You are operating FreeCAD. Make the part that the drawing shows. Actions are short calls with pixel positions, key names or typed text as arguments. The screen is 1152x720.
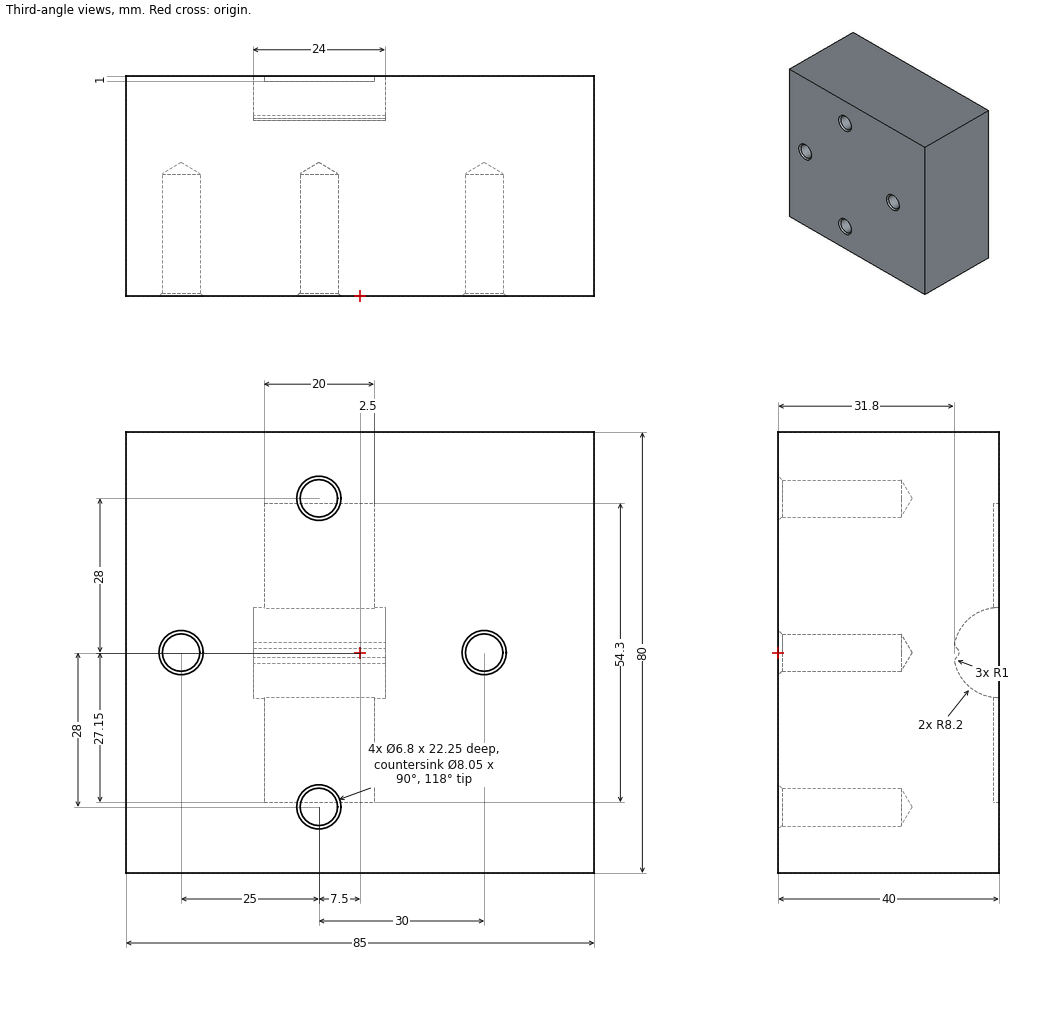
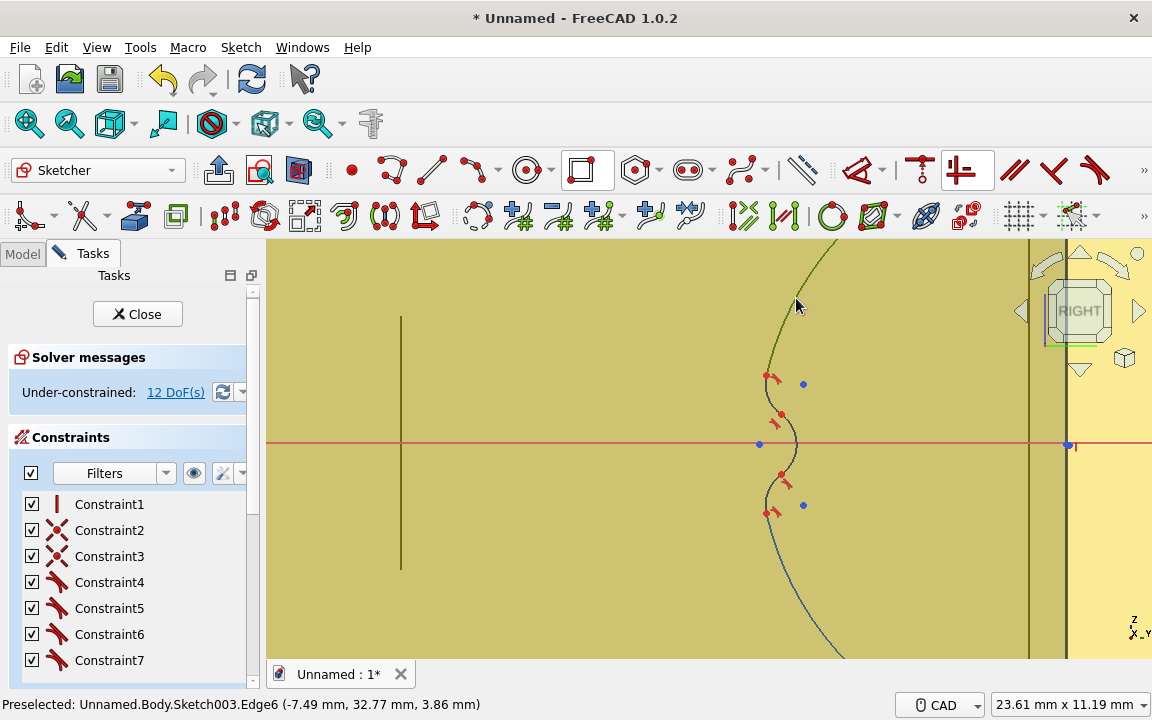
click(920, 170)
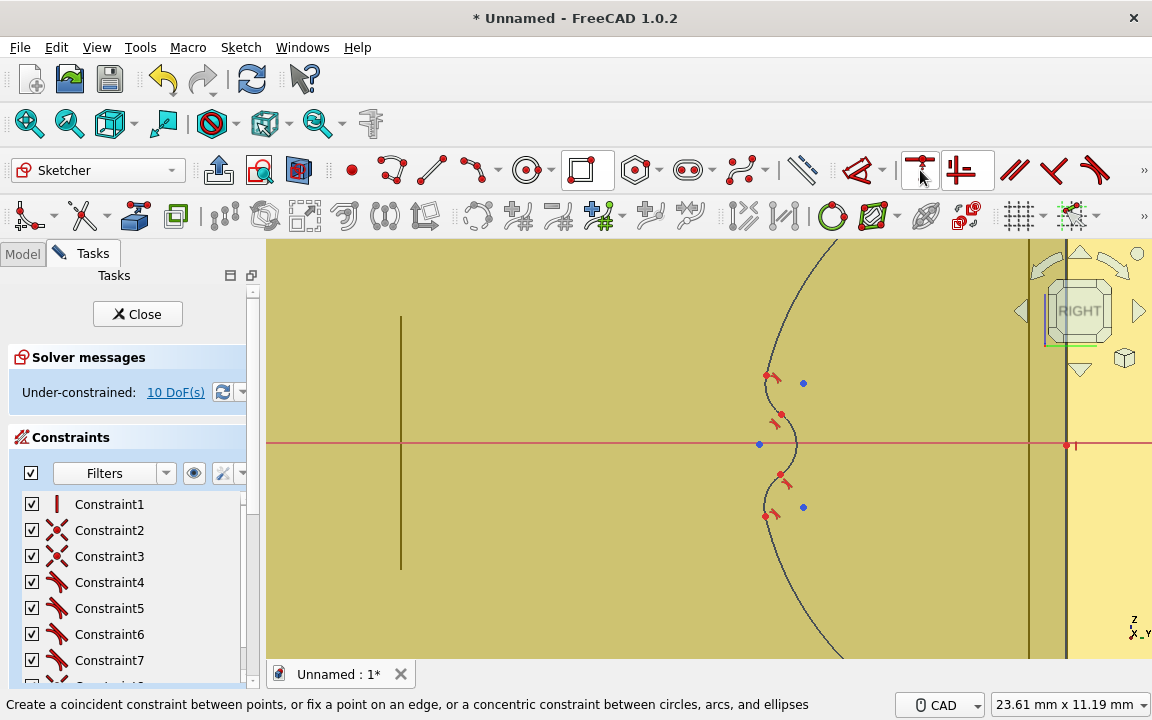
click(771, 485)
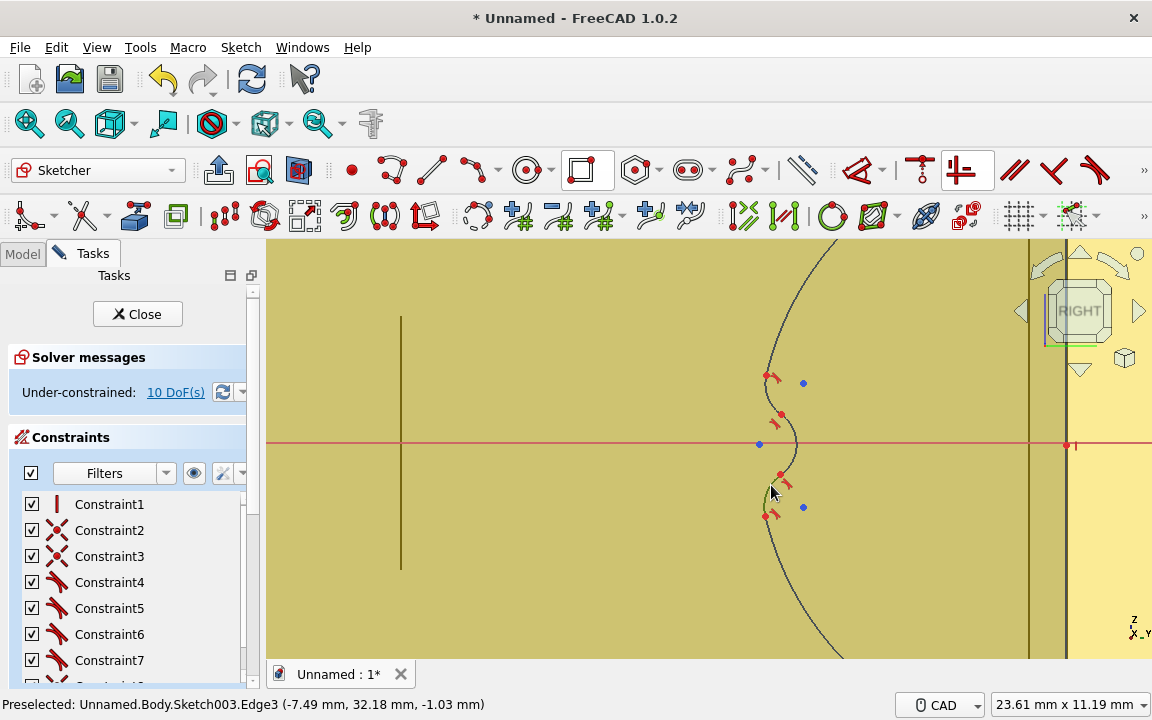
click(794, 458)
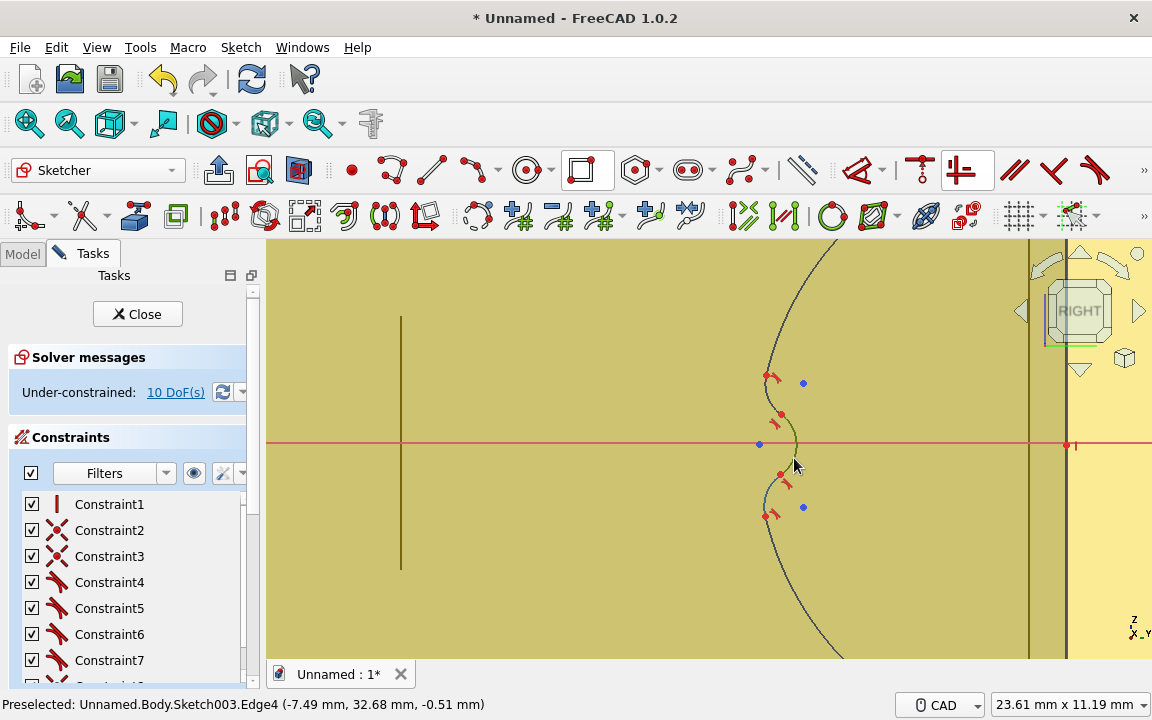
click(766, 389)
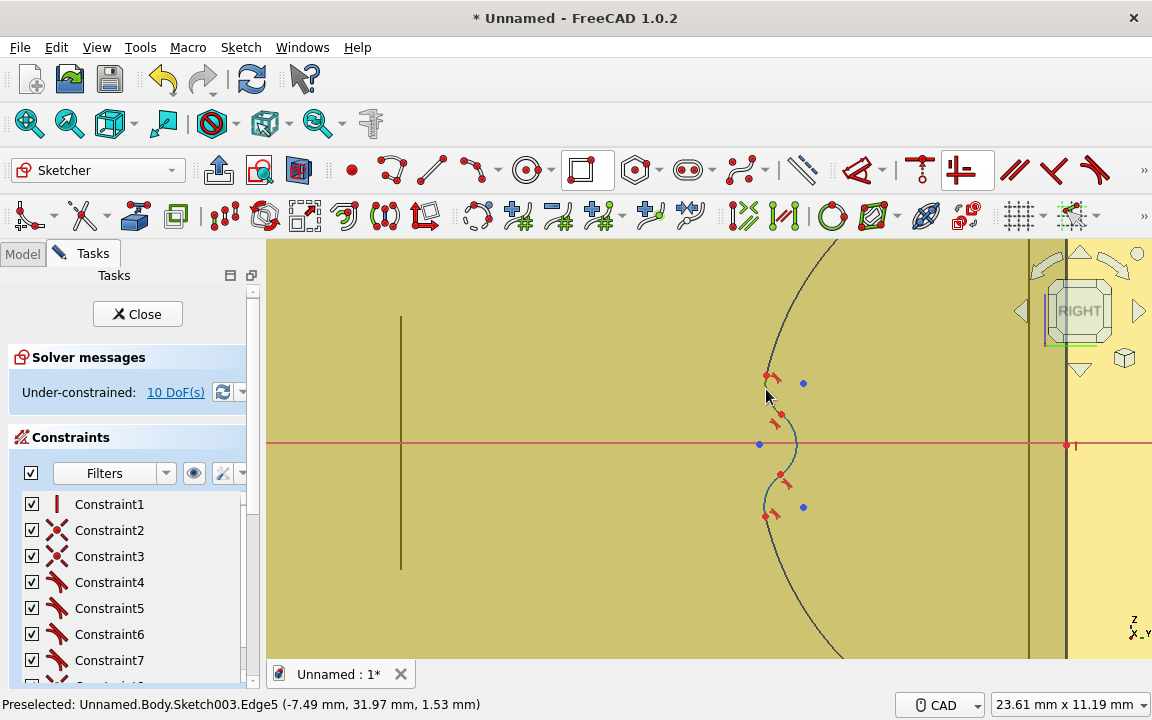
key(e)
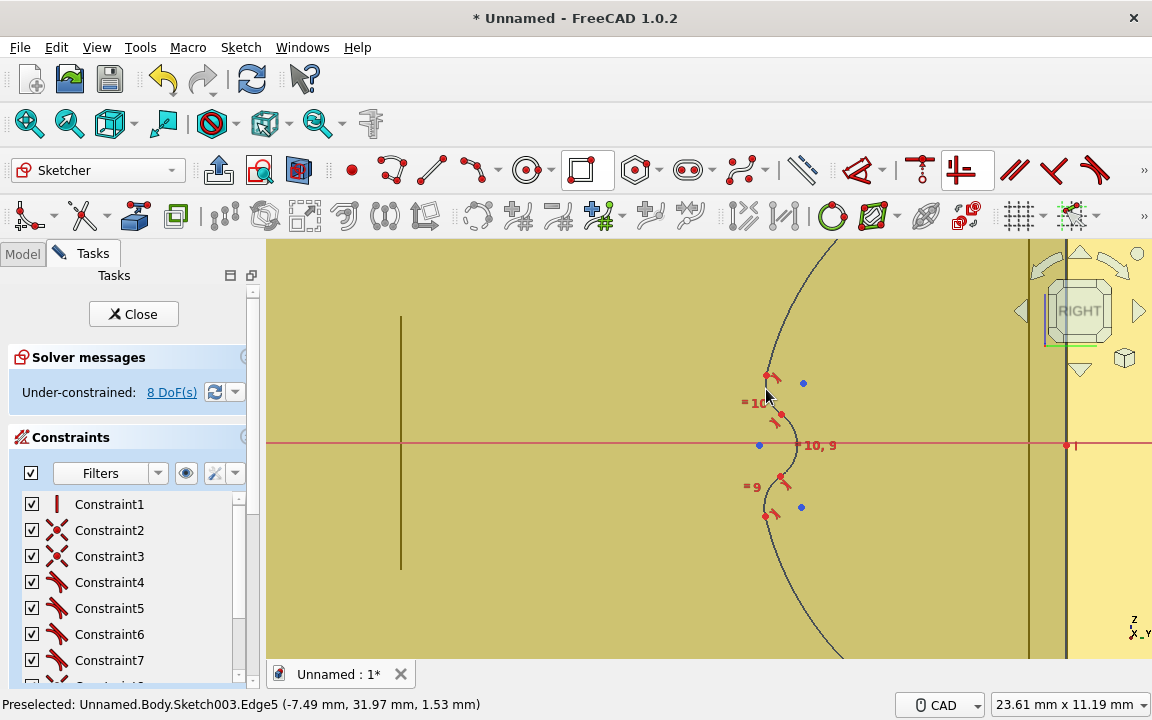
click(817, 628)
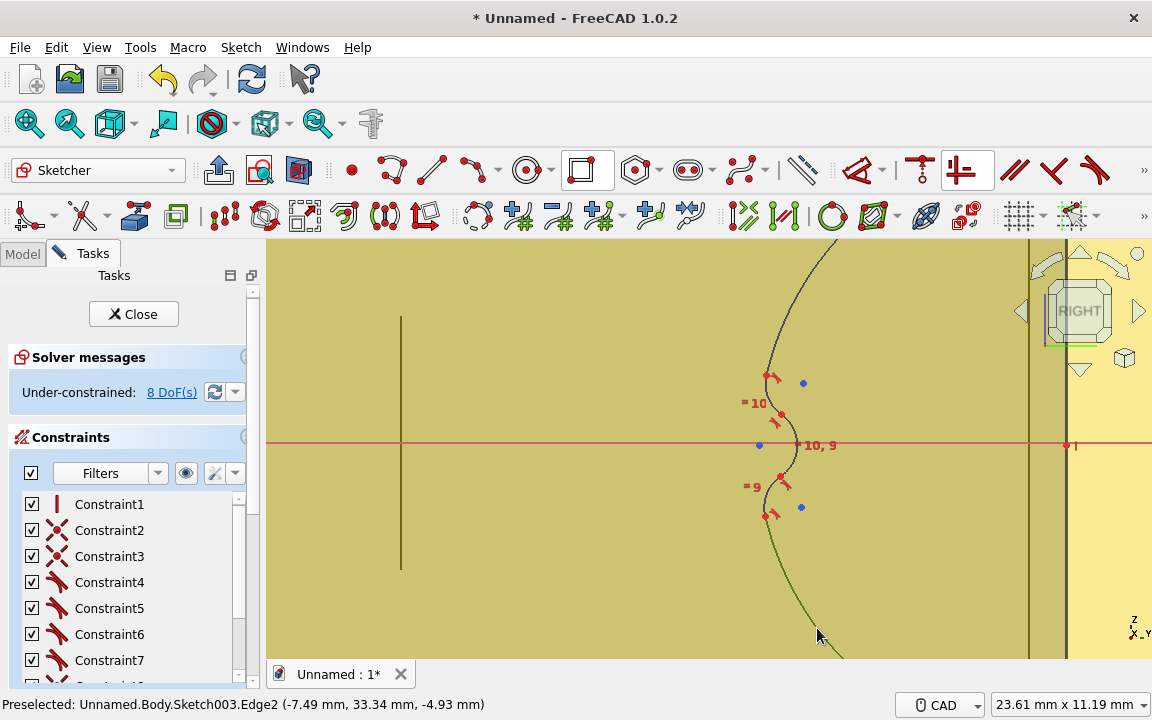
click(796, 298)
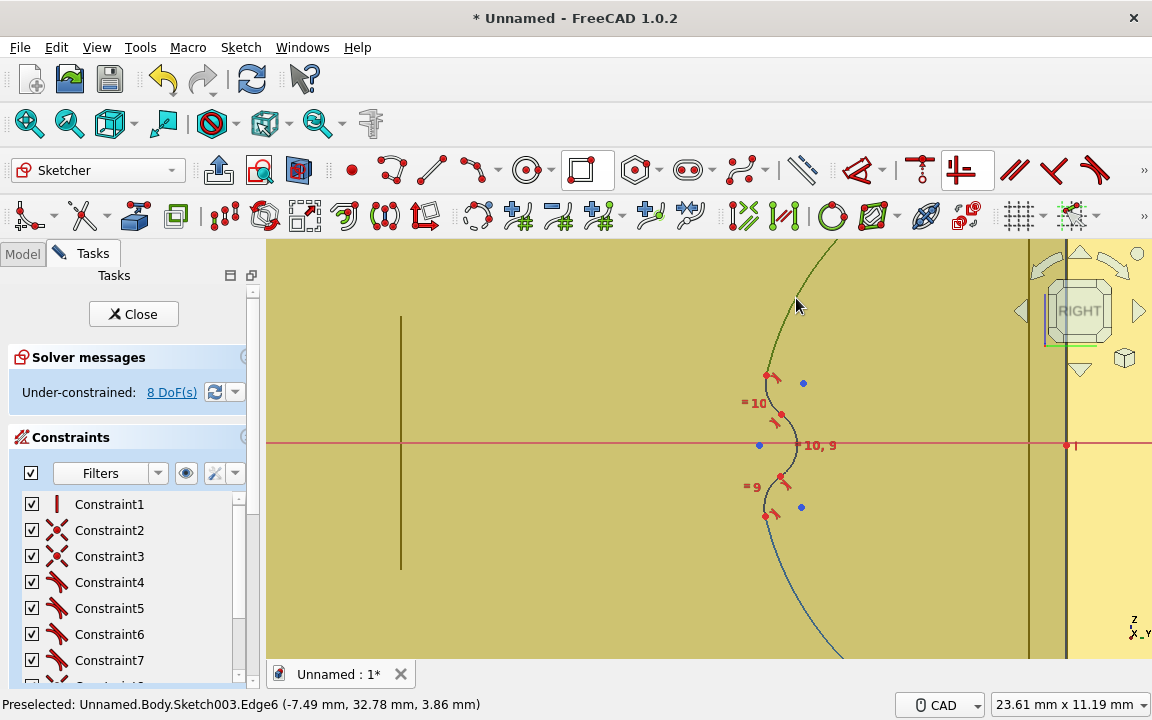
key(e)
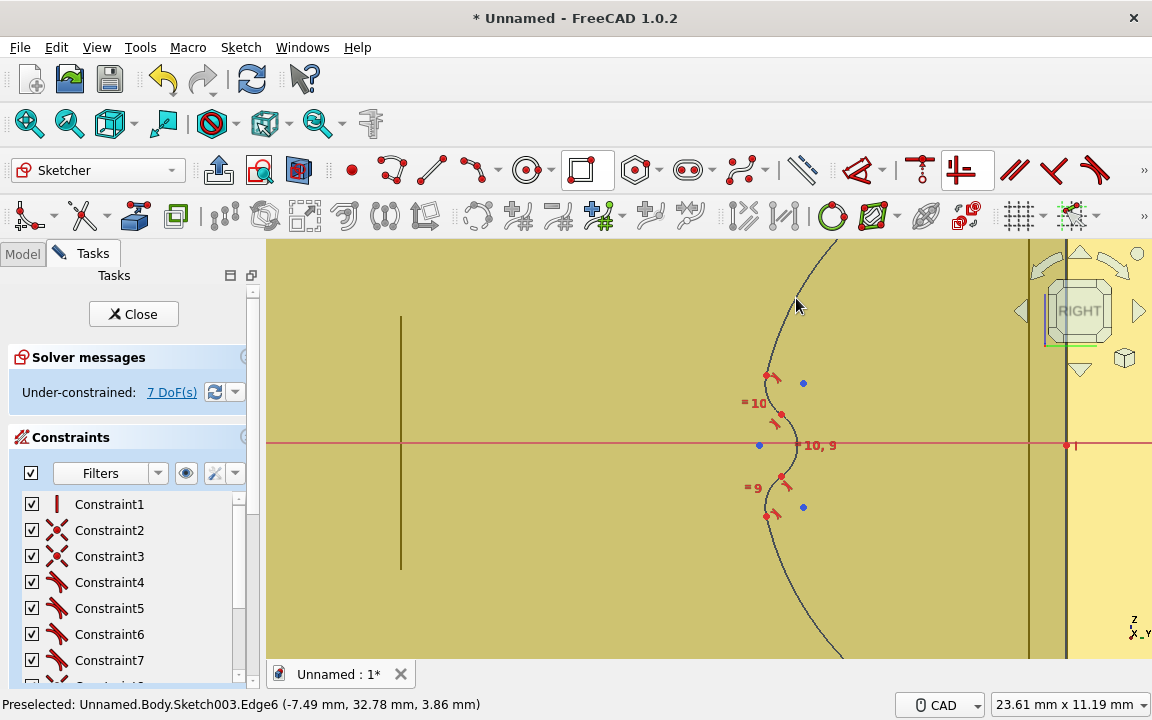
scroll(780, 451, down, 6)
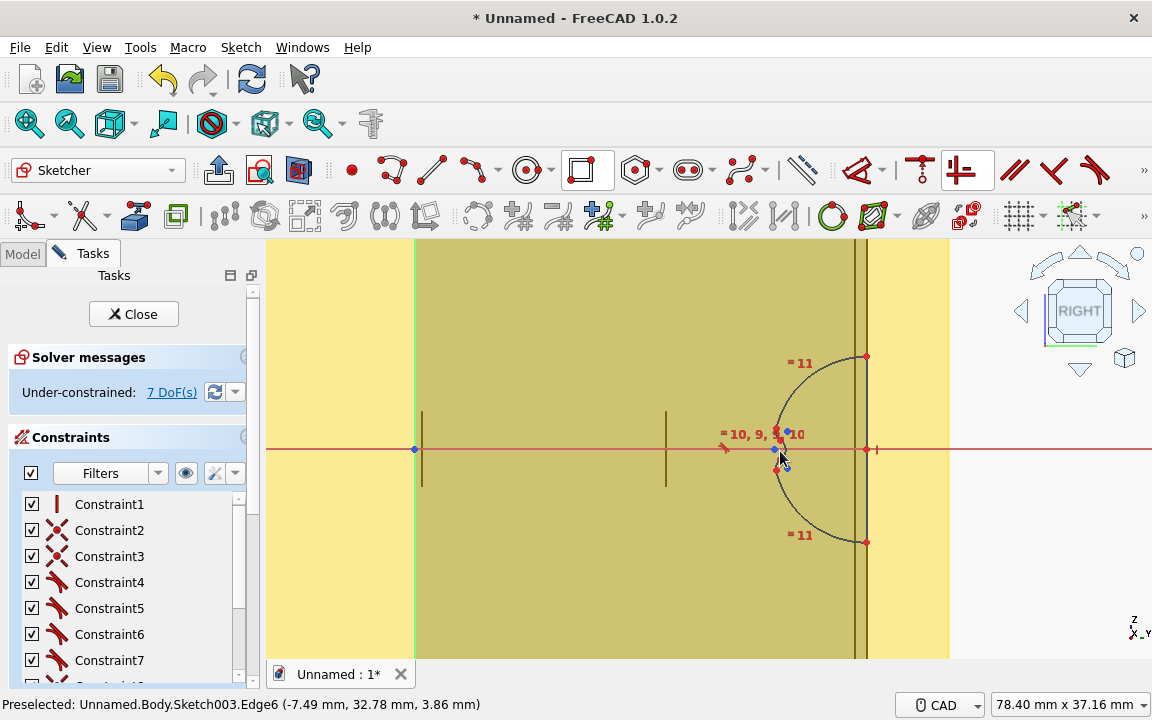
click(867, 450)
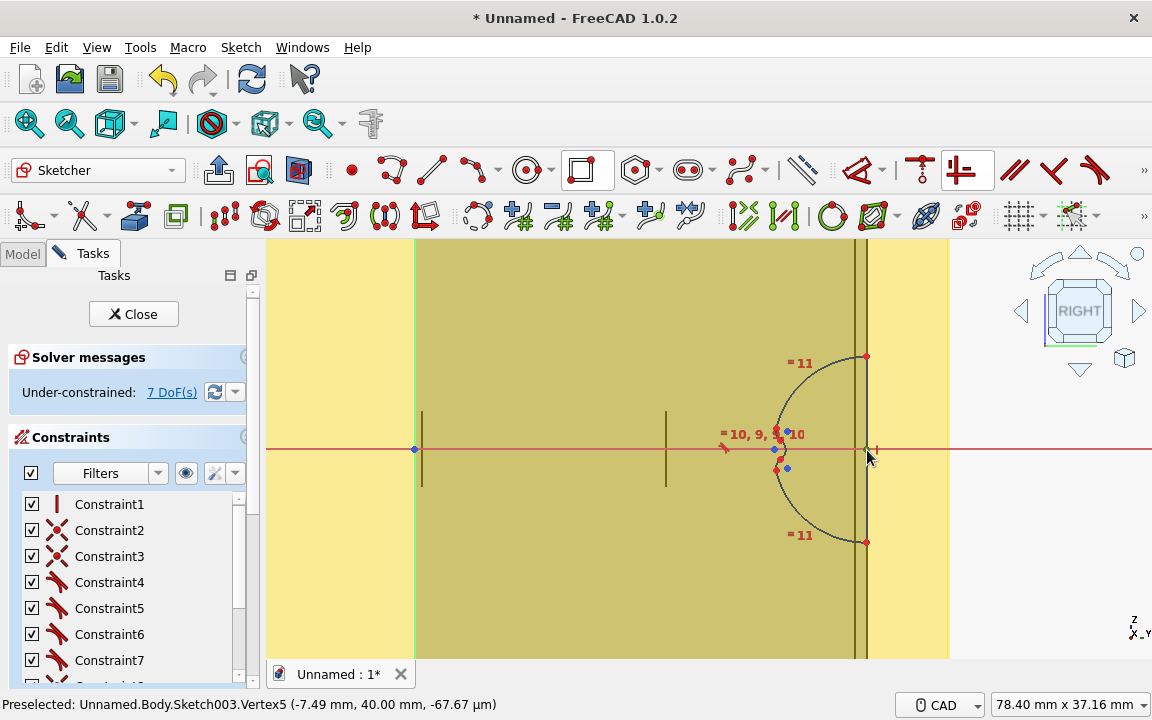
click(344, 449)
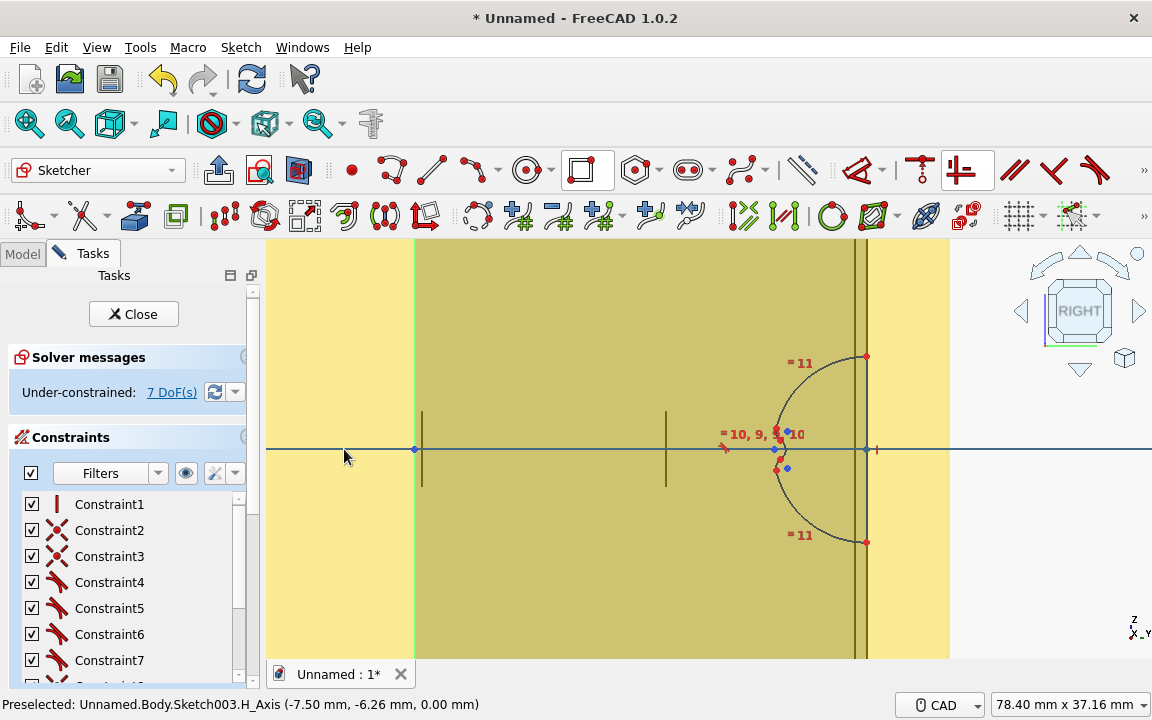
key(c)